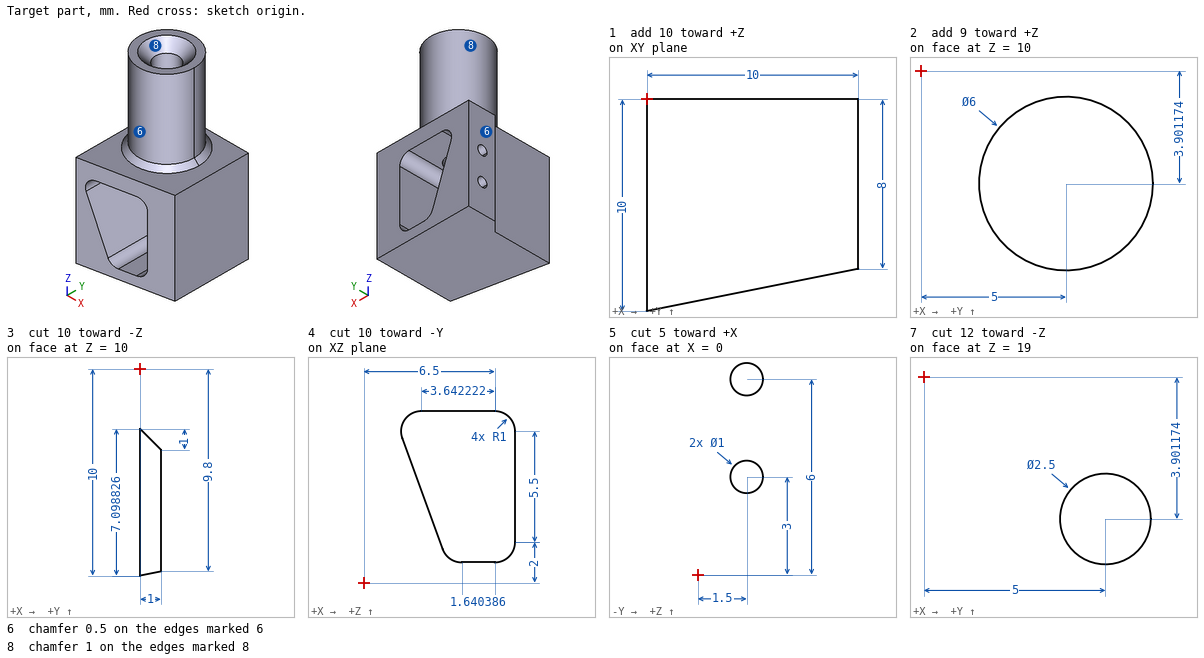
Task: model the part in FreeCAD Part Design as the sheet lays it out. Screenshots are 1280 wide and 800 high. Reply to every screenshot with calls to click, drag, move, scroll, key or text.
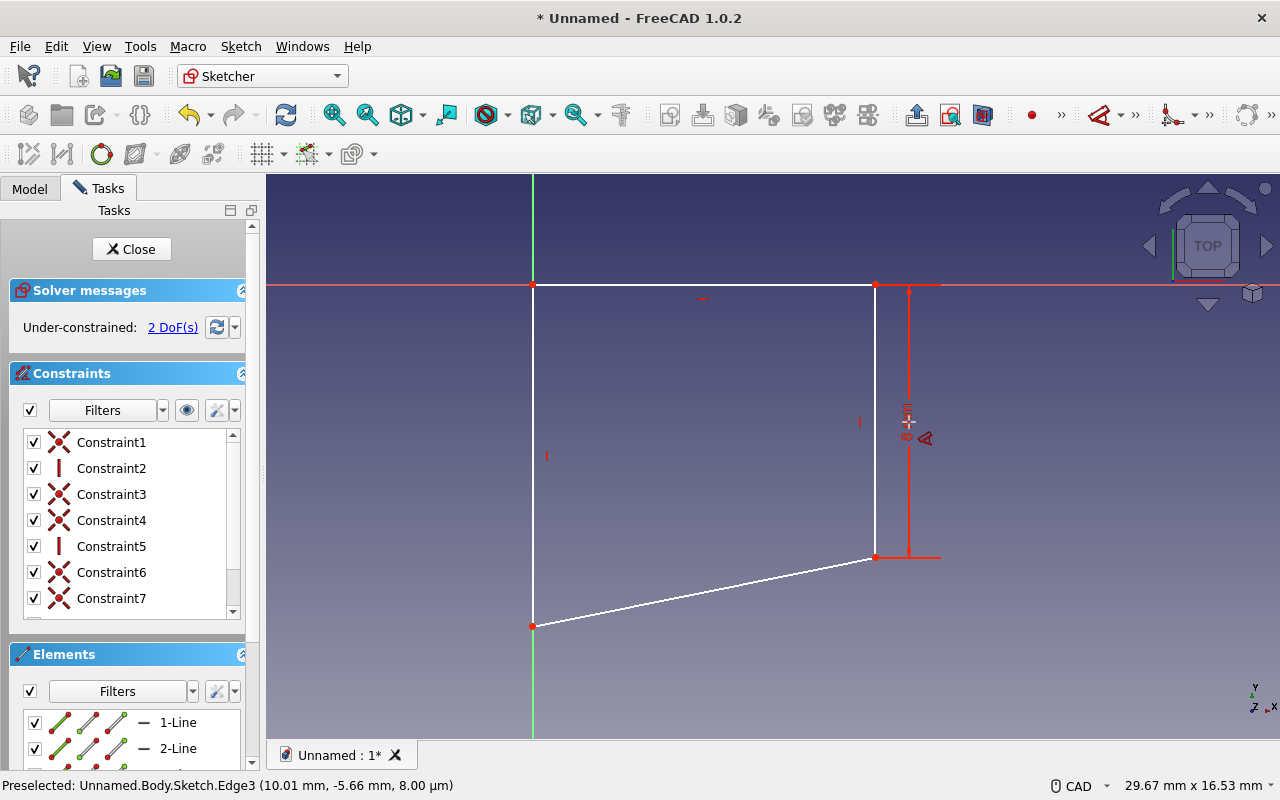
click(533, 387)
click(499, 456)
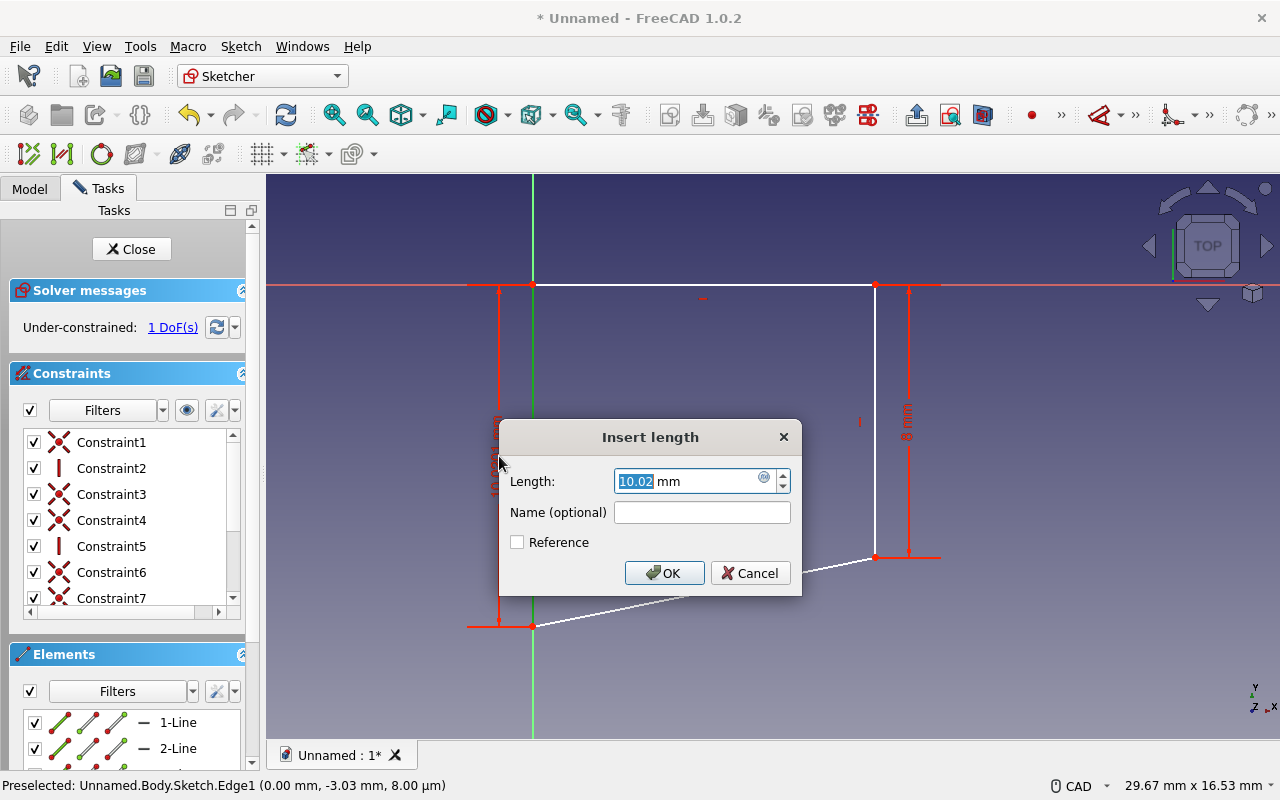
text(10)
key(Return)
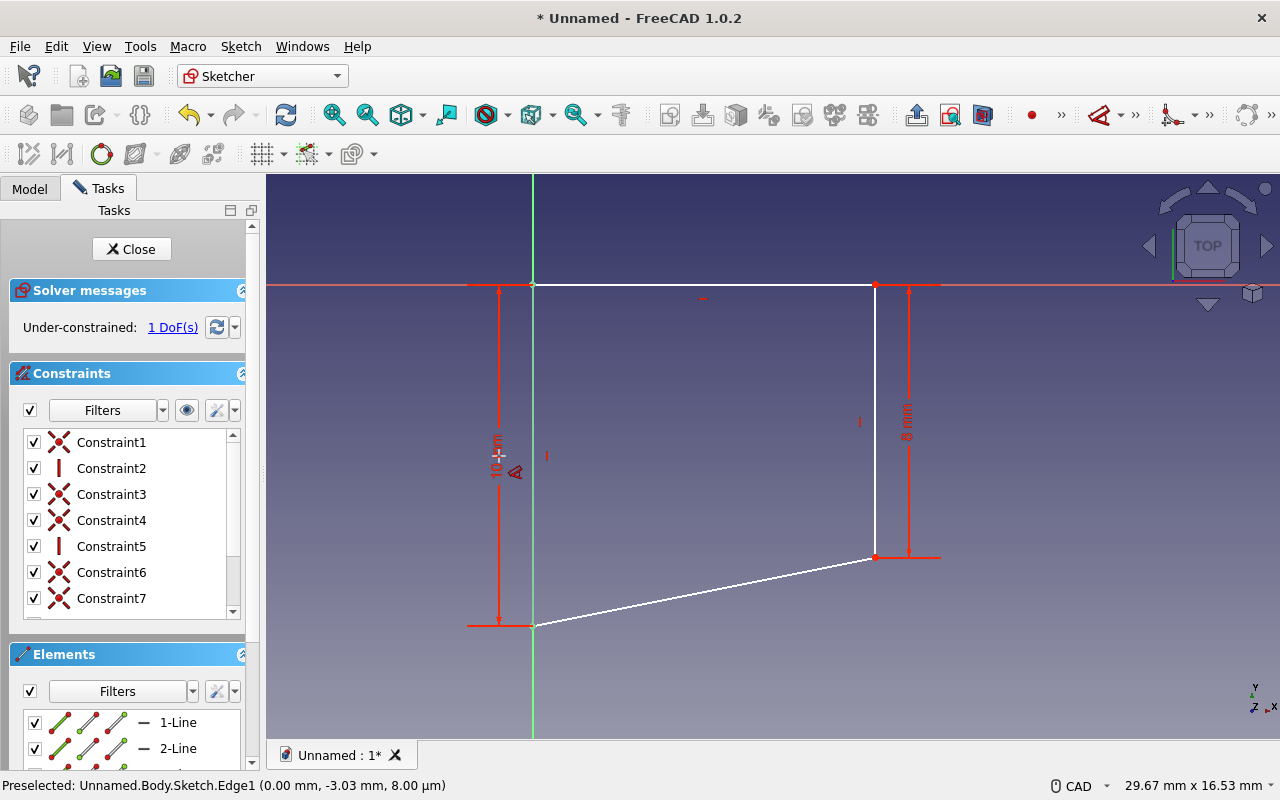
click(772, 285)
click(704, 251)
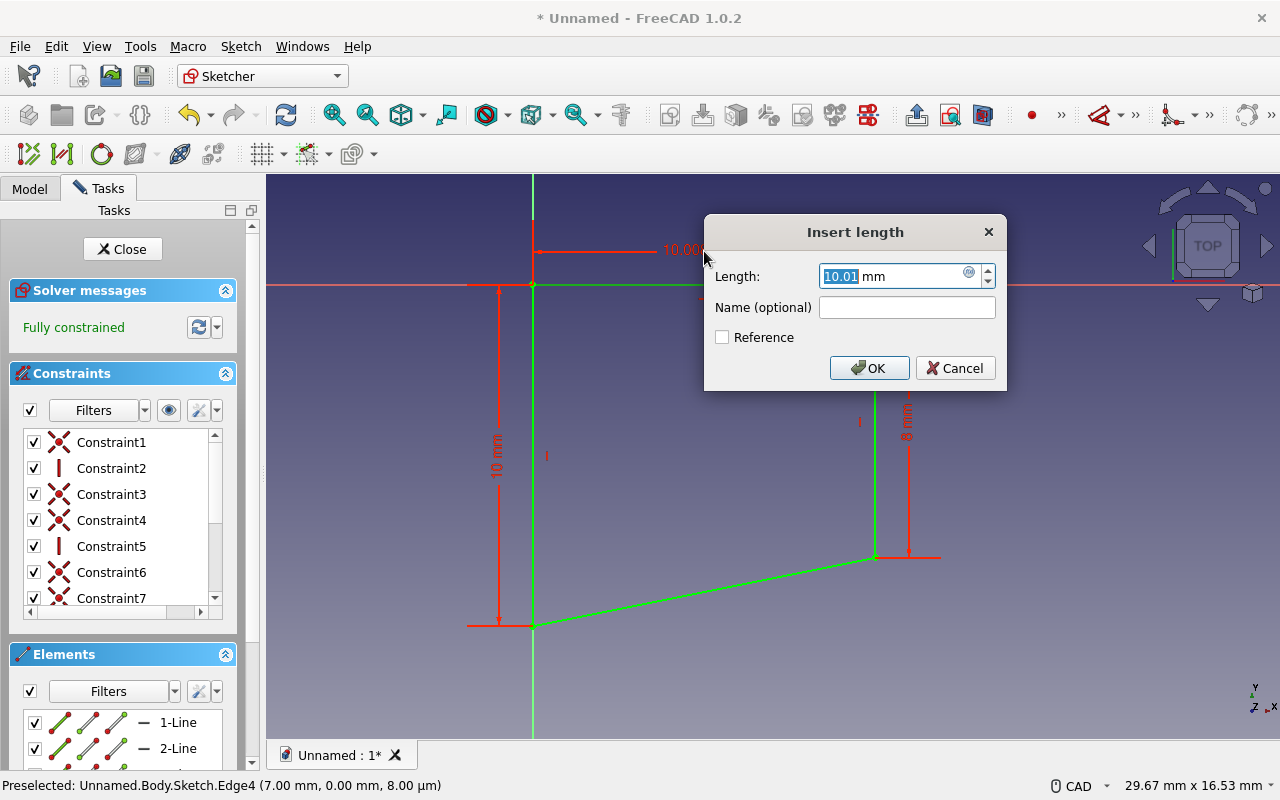
text(10)
key(Return)
key(Escape)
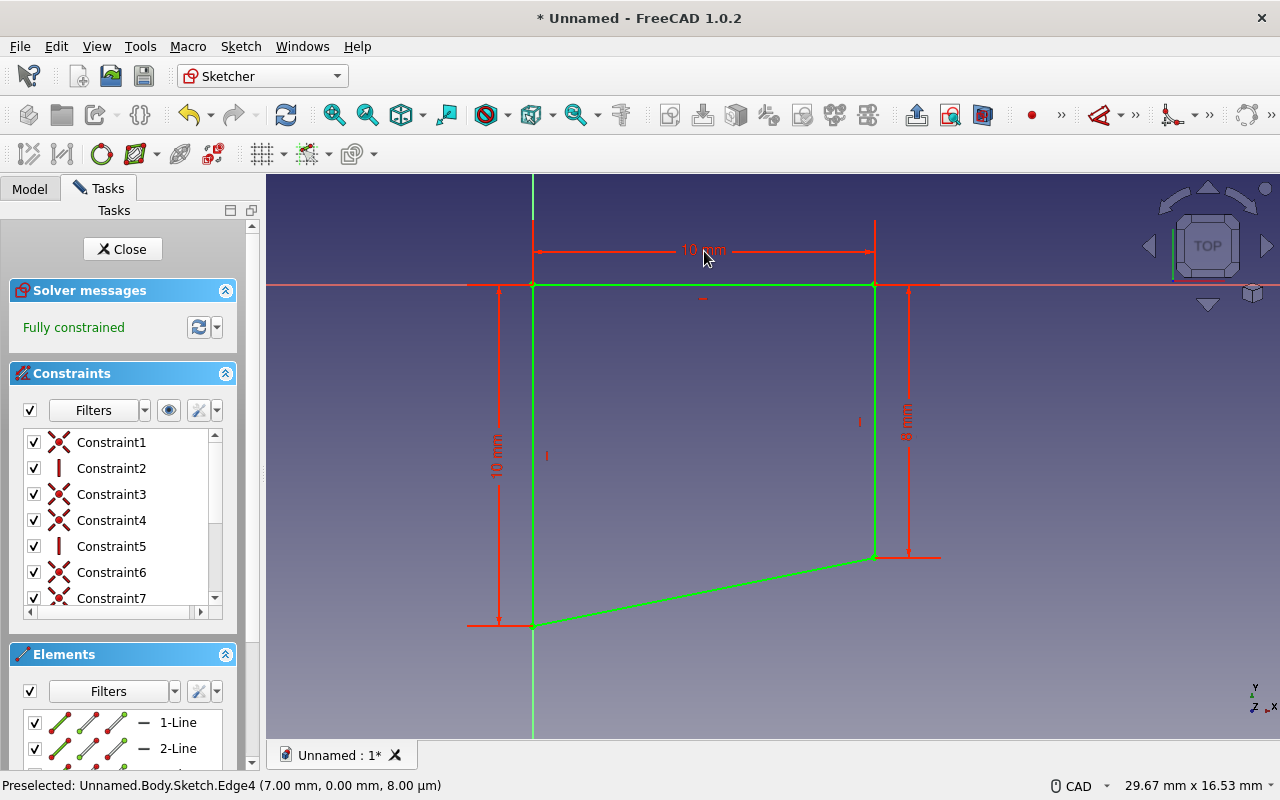
click(123, 249)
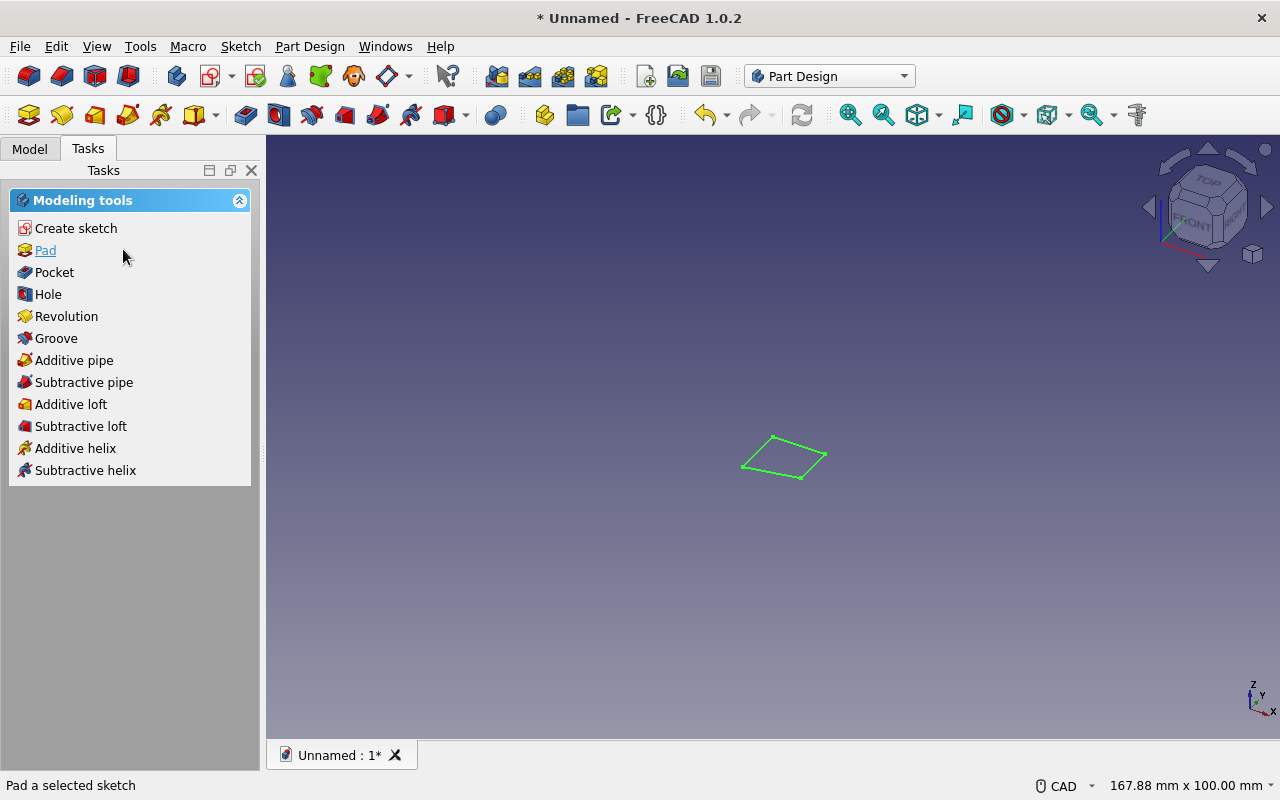
click(29, 116)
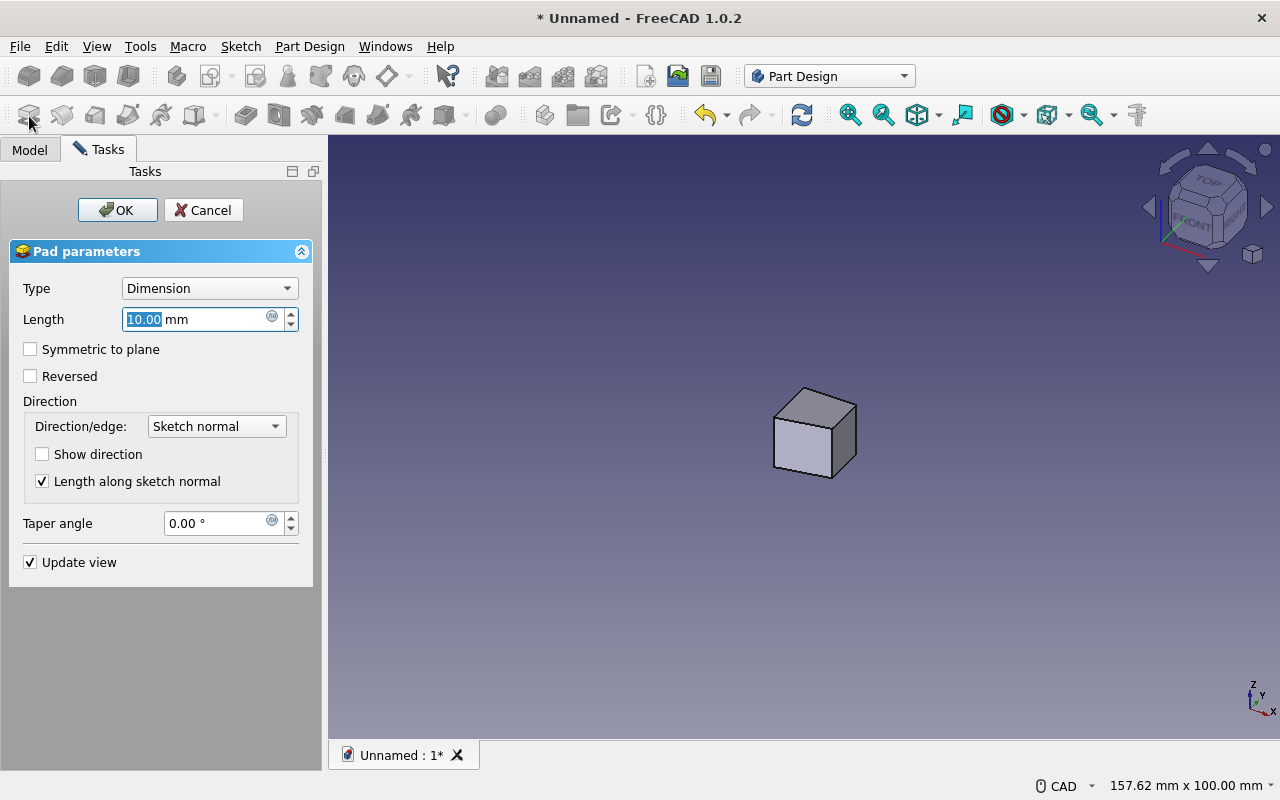
text(10)
key(Tab)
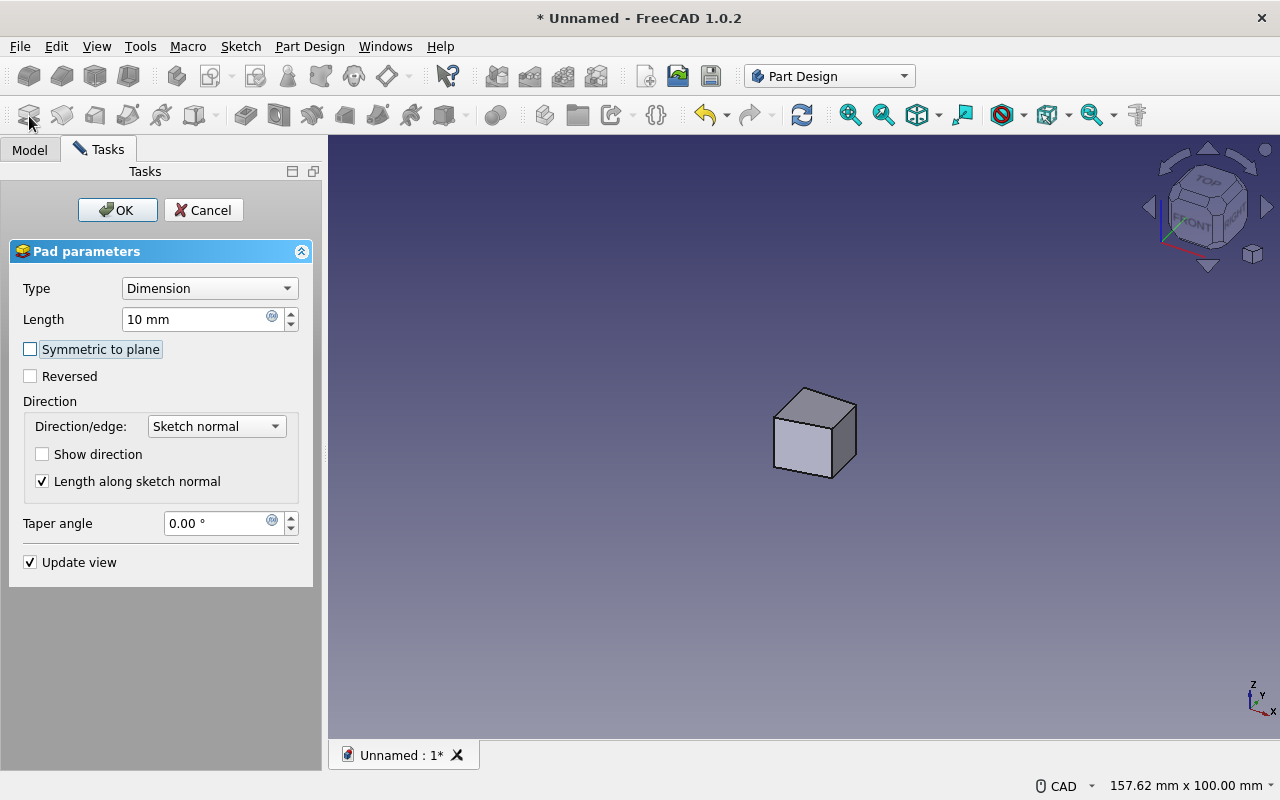
click(118, 210)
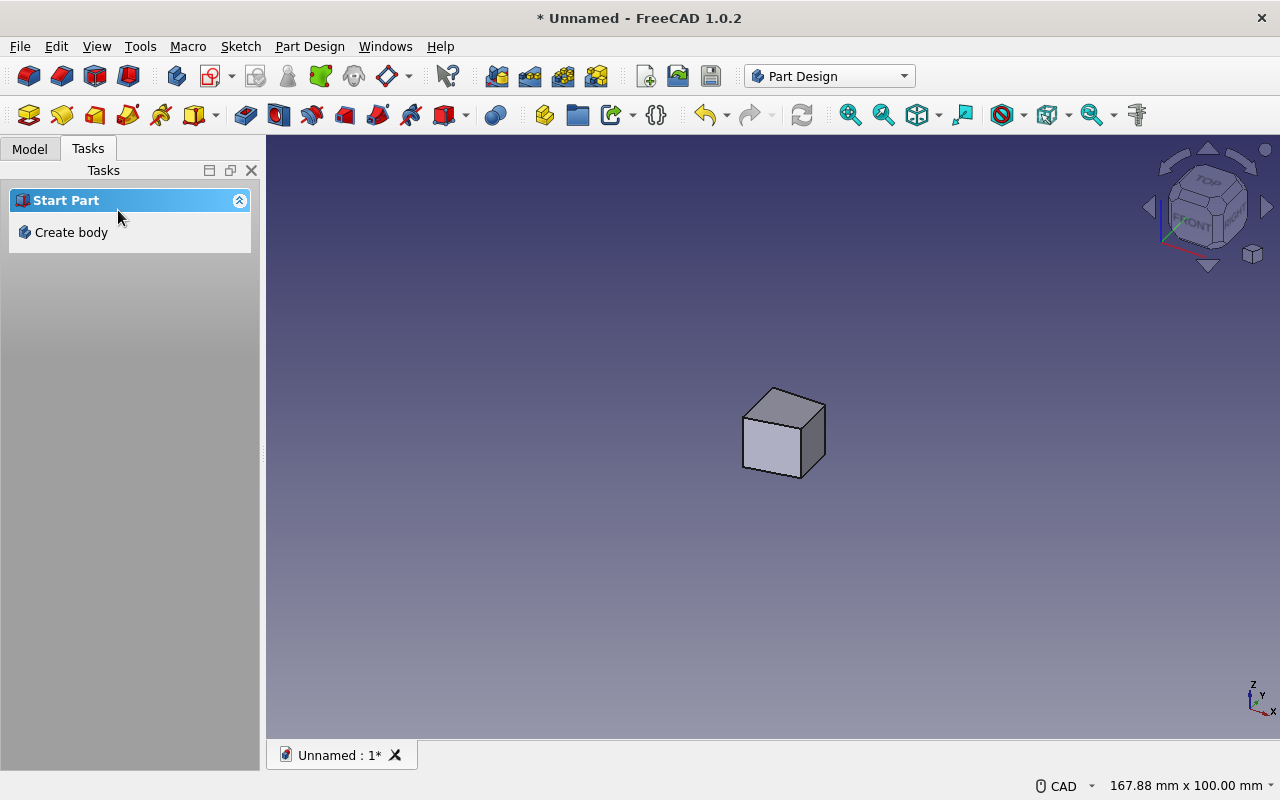
key(v)
key(f)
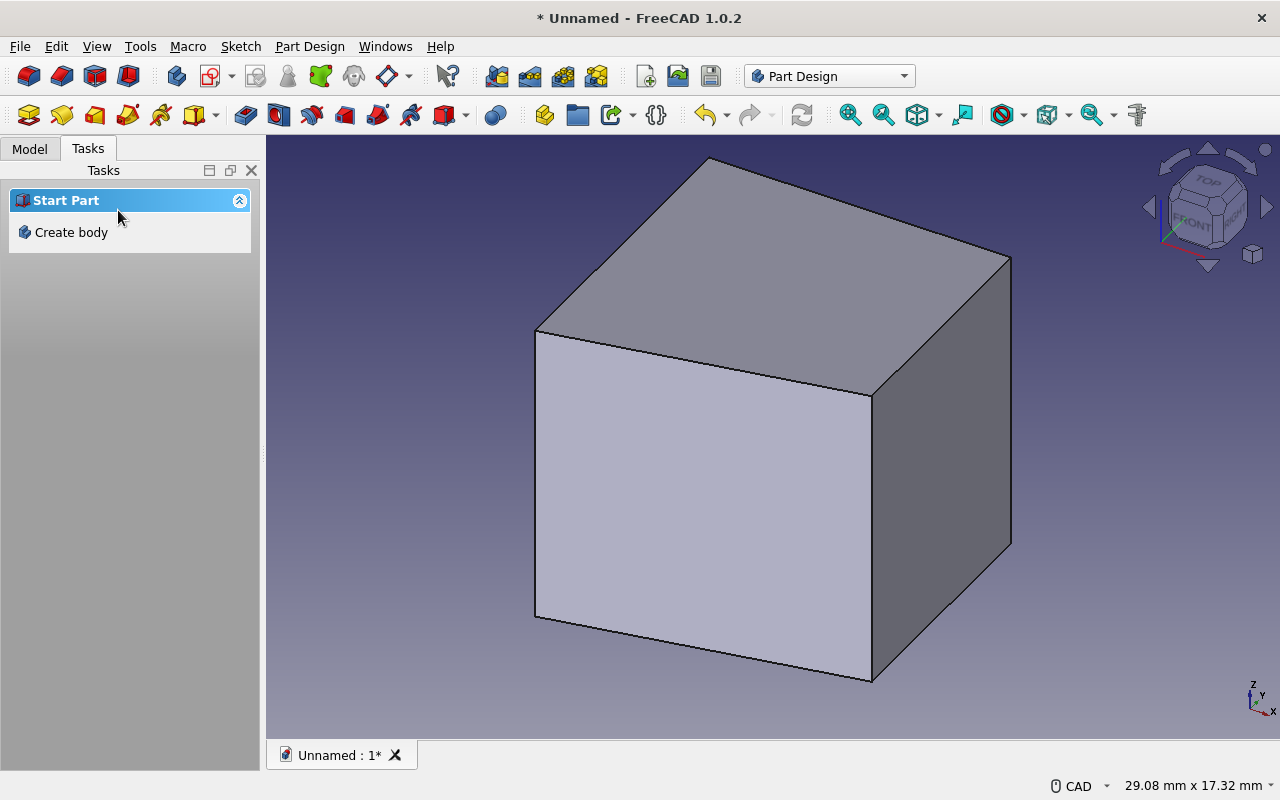
click(773, 293)